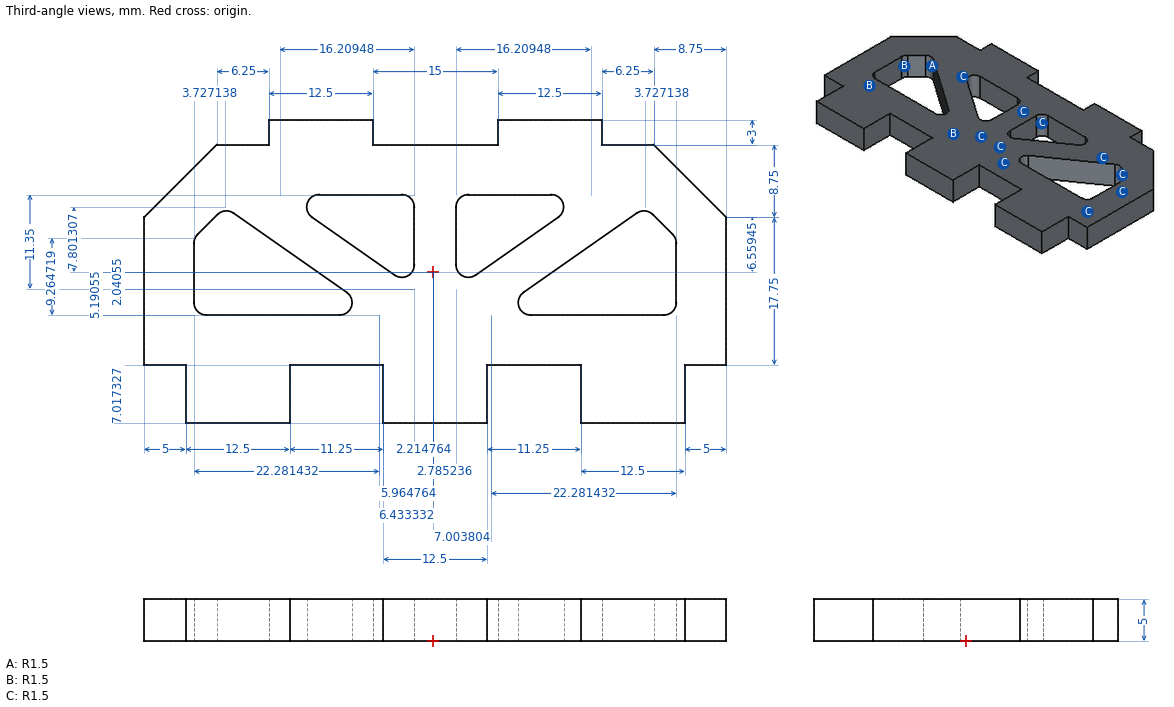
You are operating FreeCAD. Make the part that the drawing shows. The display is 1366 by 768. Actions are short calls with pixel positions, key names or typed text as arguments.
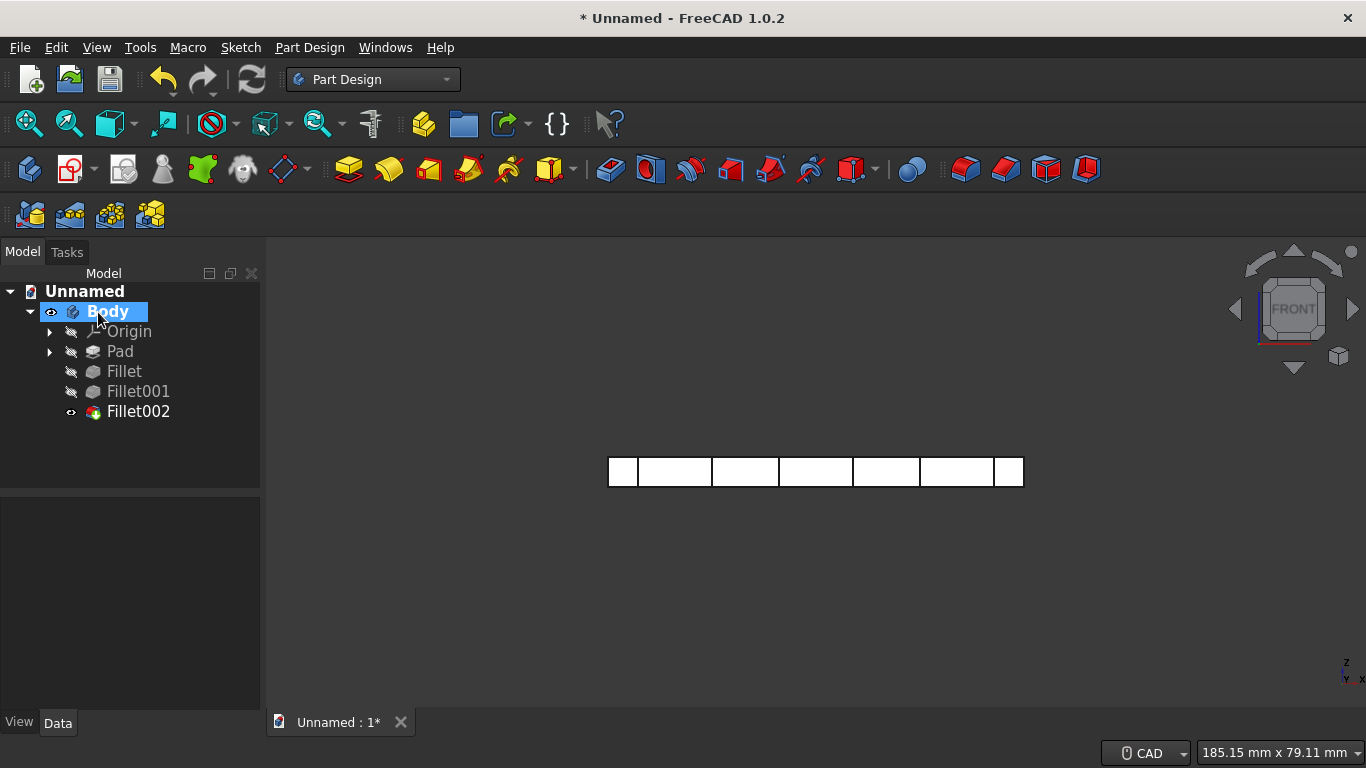
key(0)